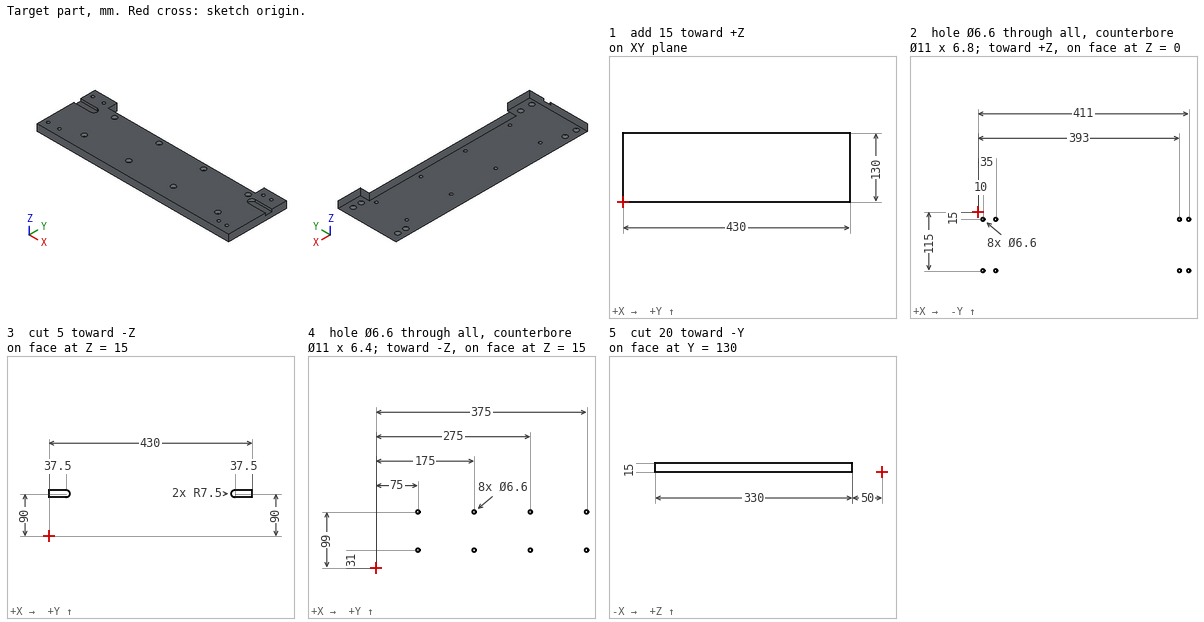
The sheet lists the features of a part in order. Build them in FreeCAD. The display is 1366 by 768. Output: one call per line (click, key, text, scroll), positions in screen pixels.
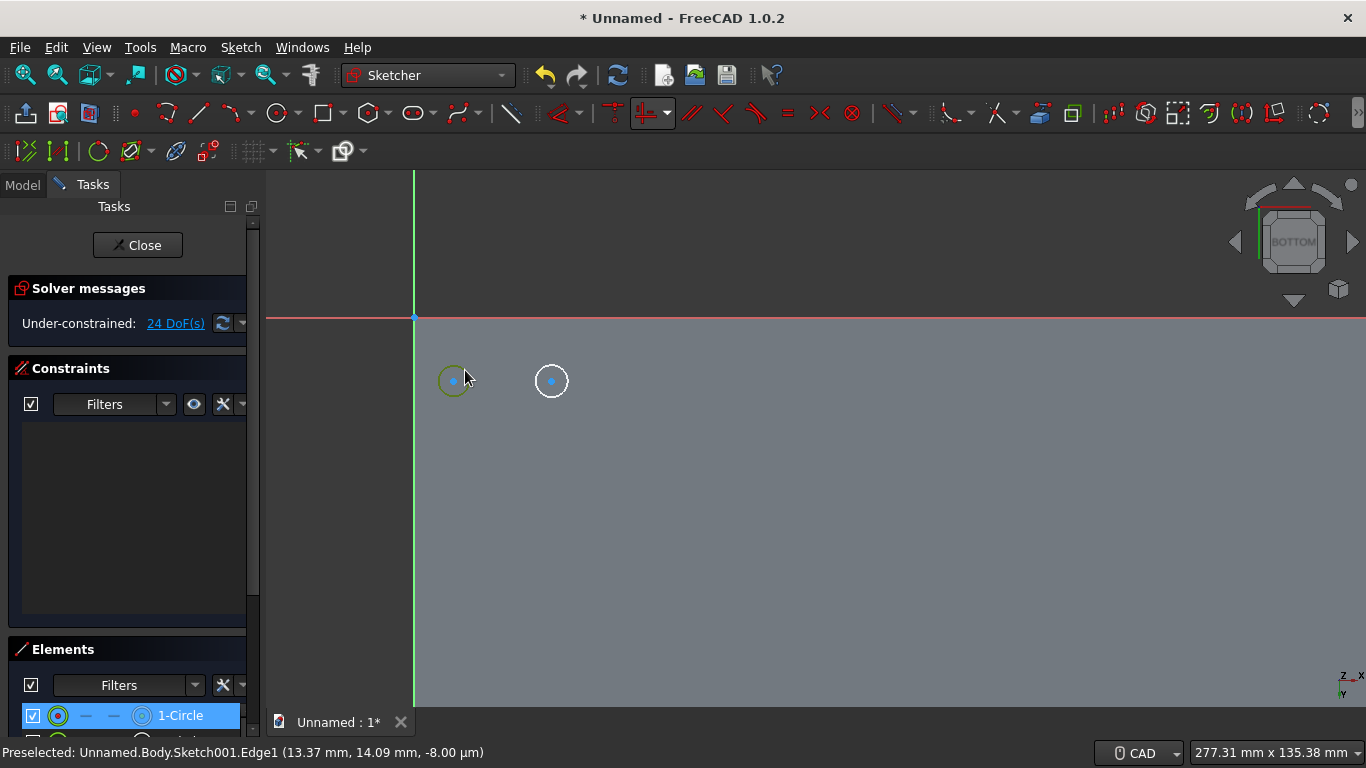
scroll(463, 372, down, 5)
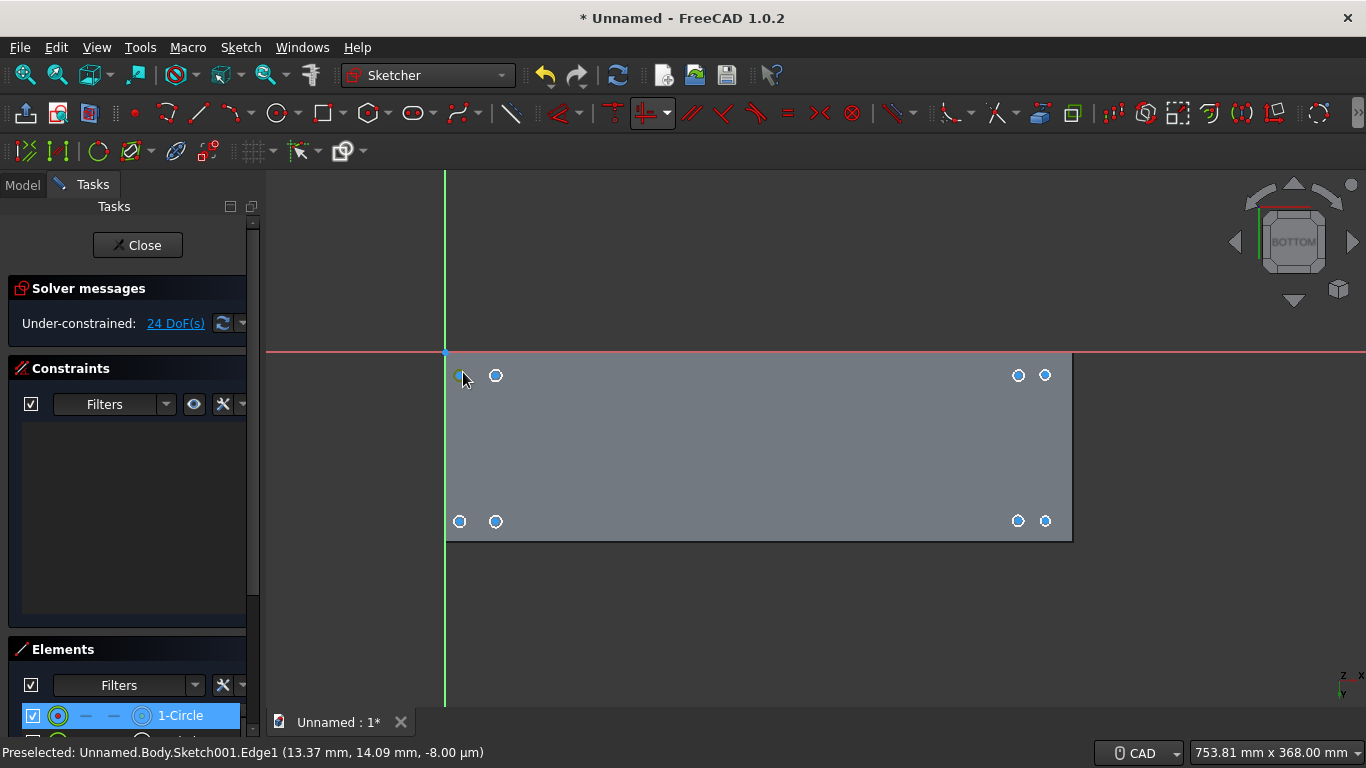
scroll(464, 518, up, 5)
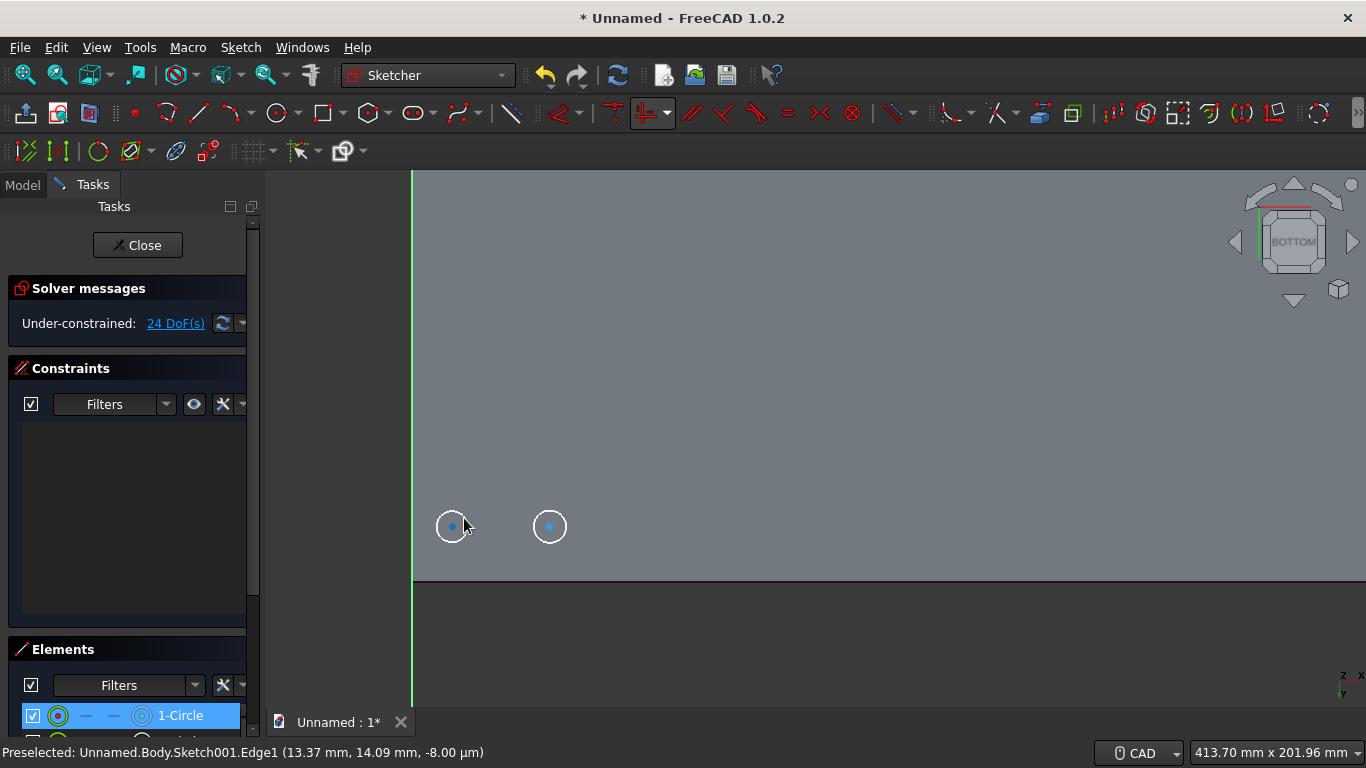
click(463, 516)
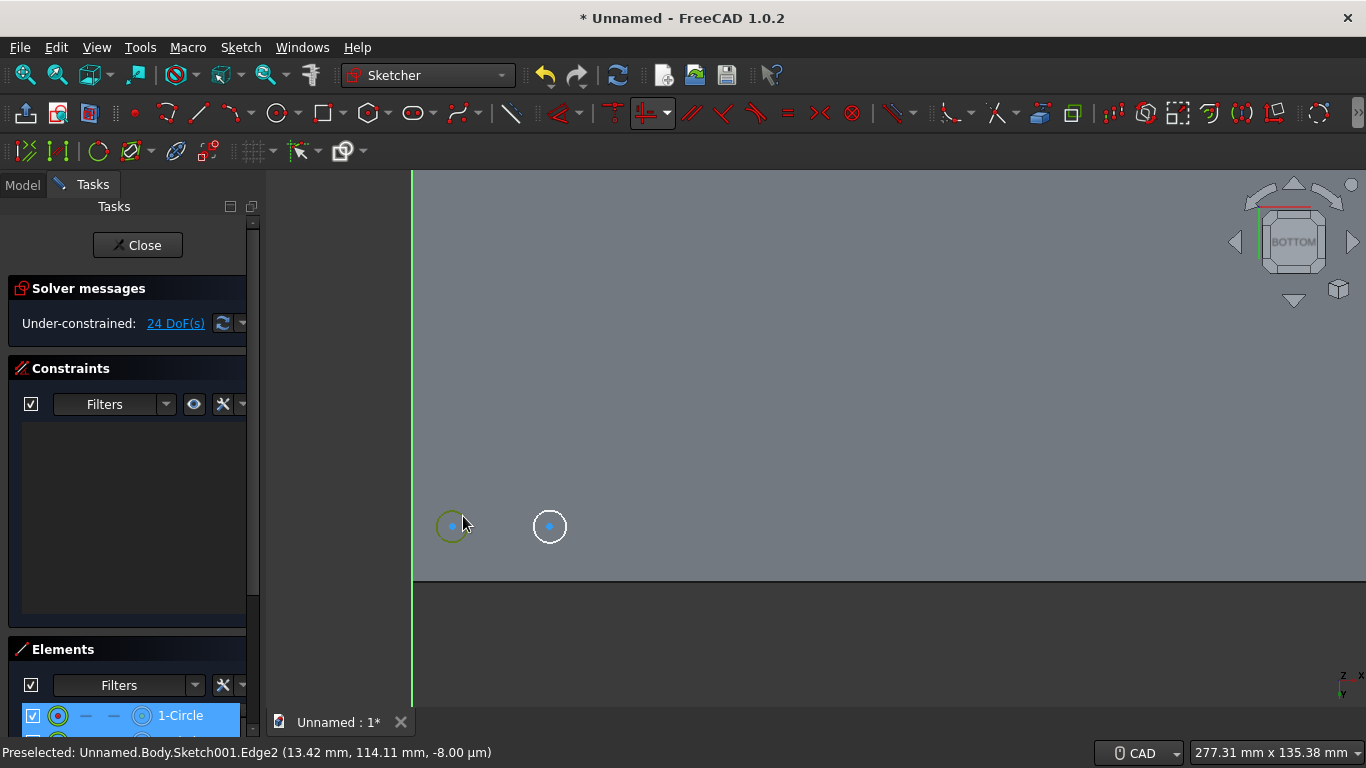
scroll(464, 518, down, 5)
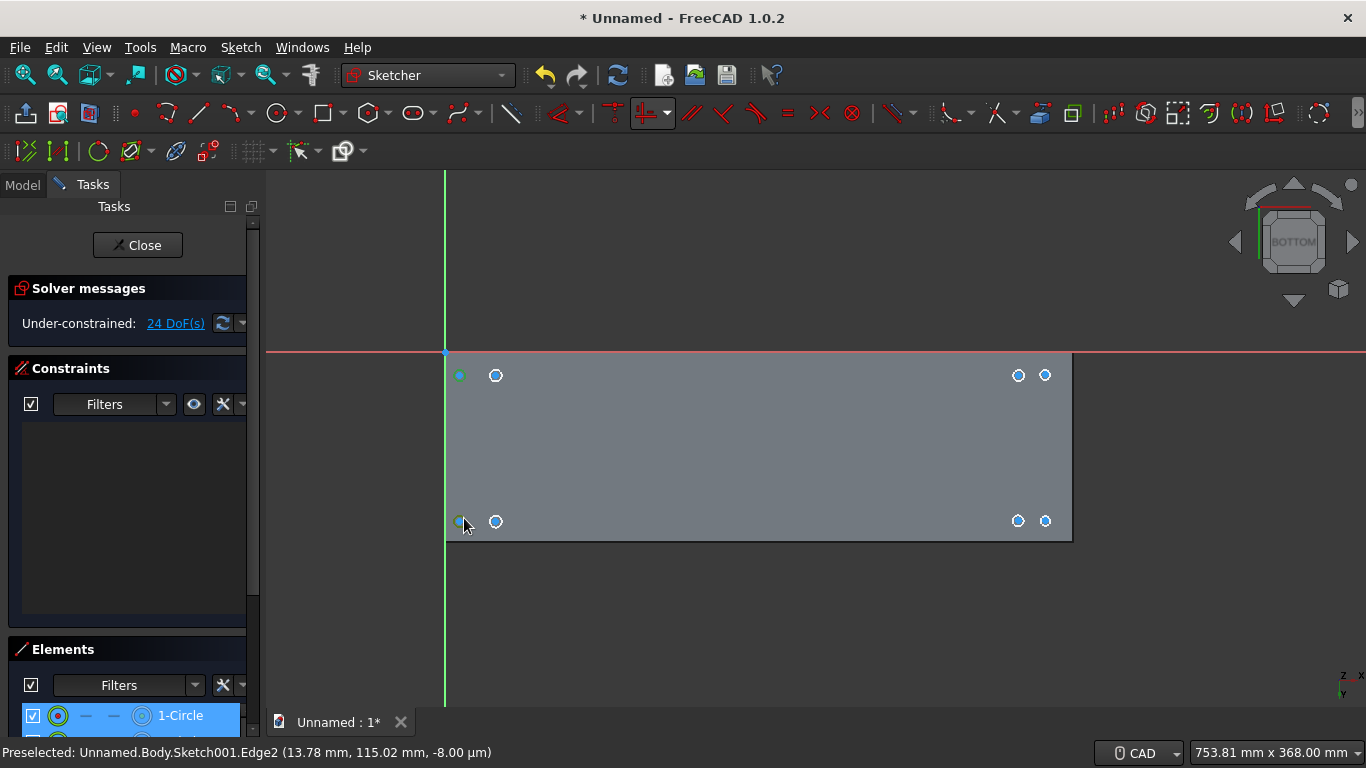
scroll(500, 371, up, 5)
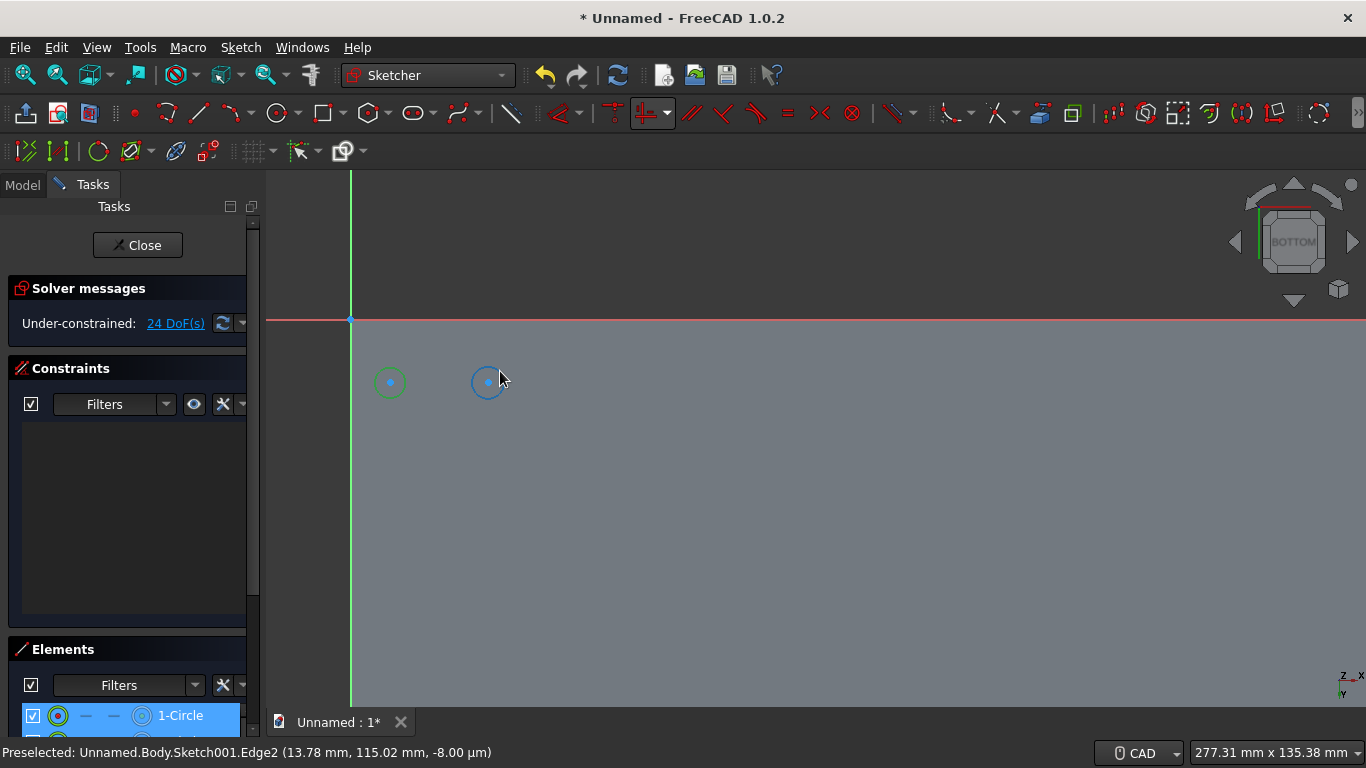
click(499, 372)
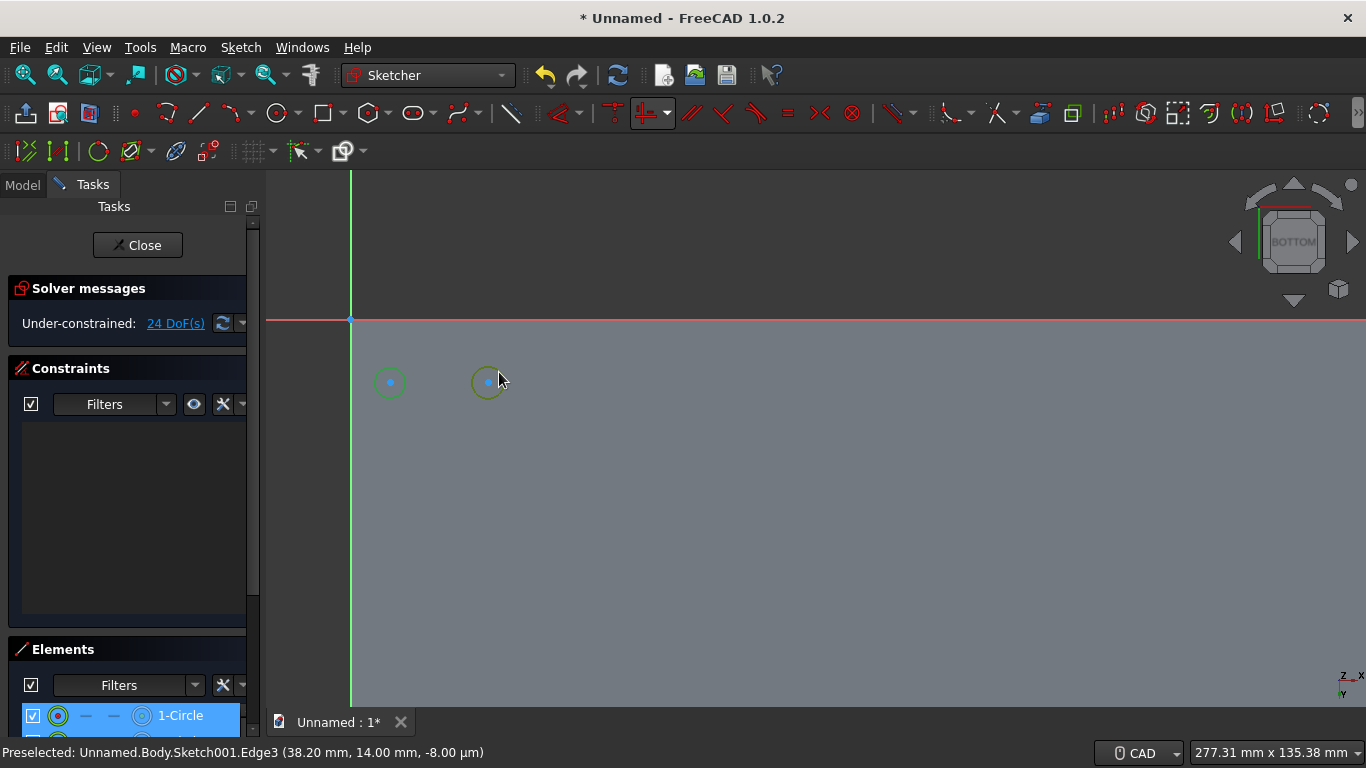
scroll(500, 371, down, 5)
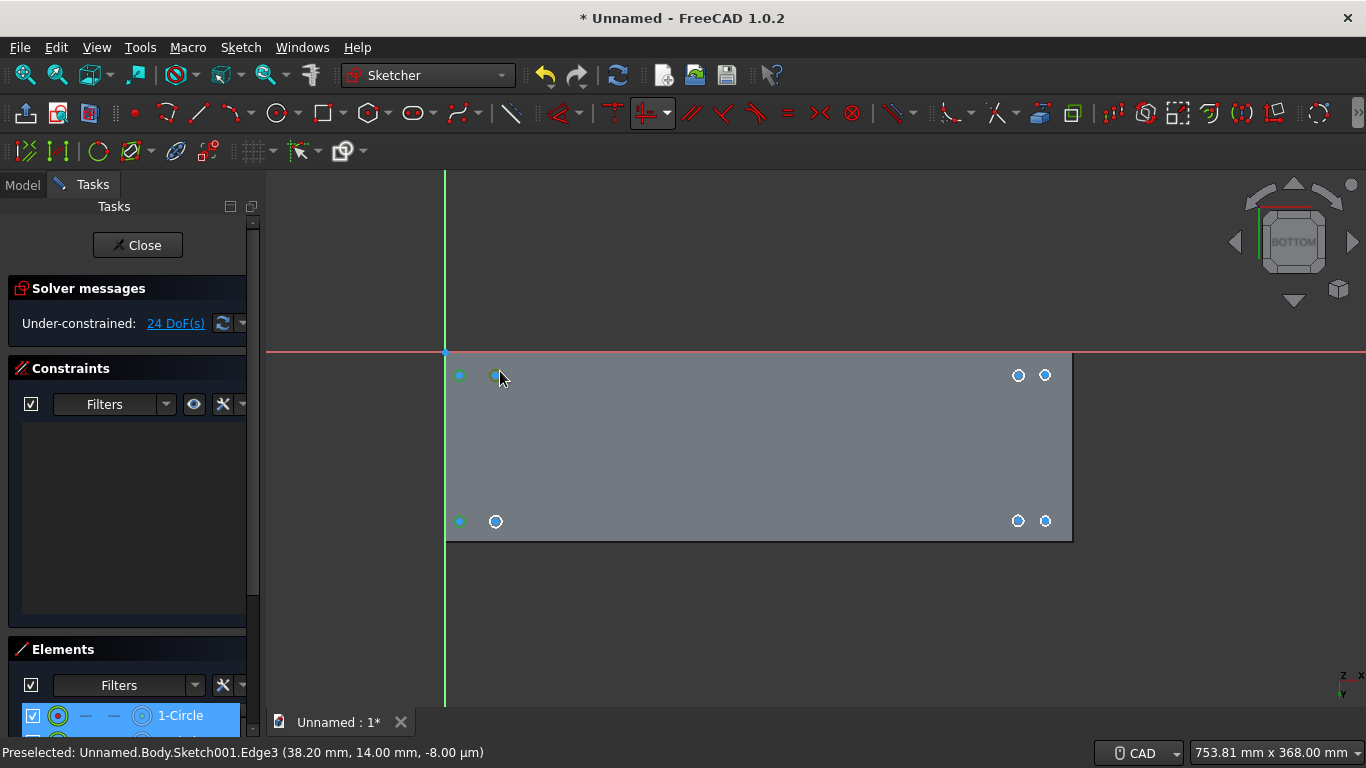
scroll(500, 517, up, 5)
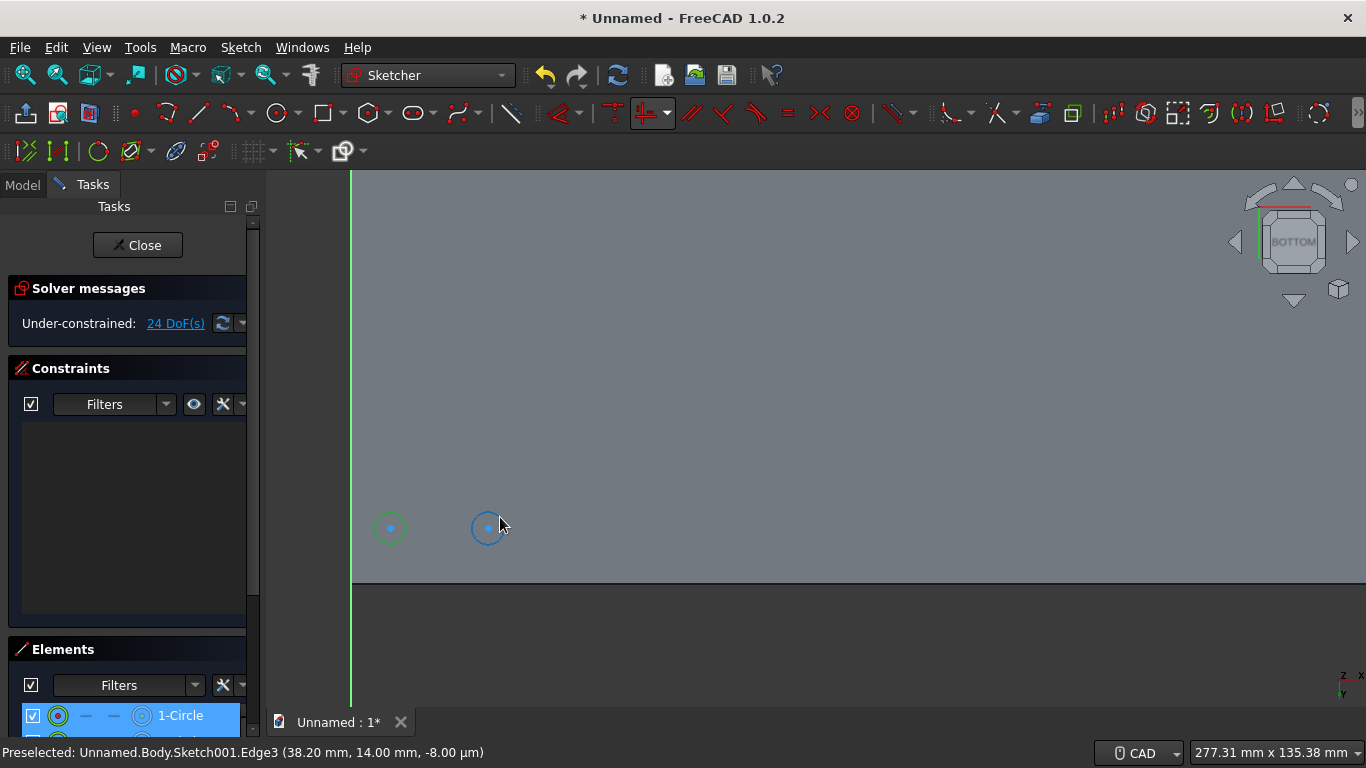
click(499, 517)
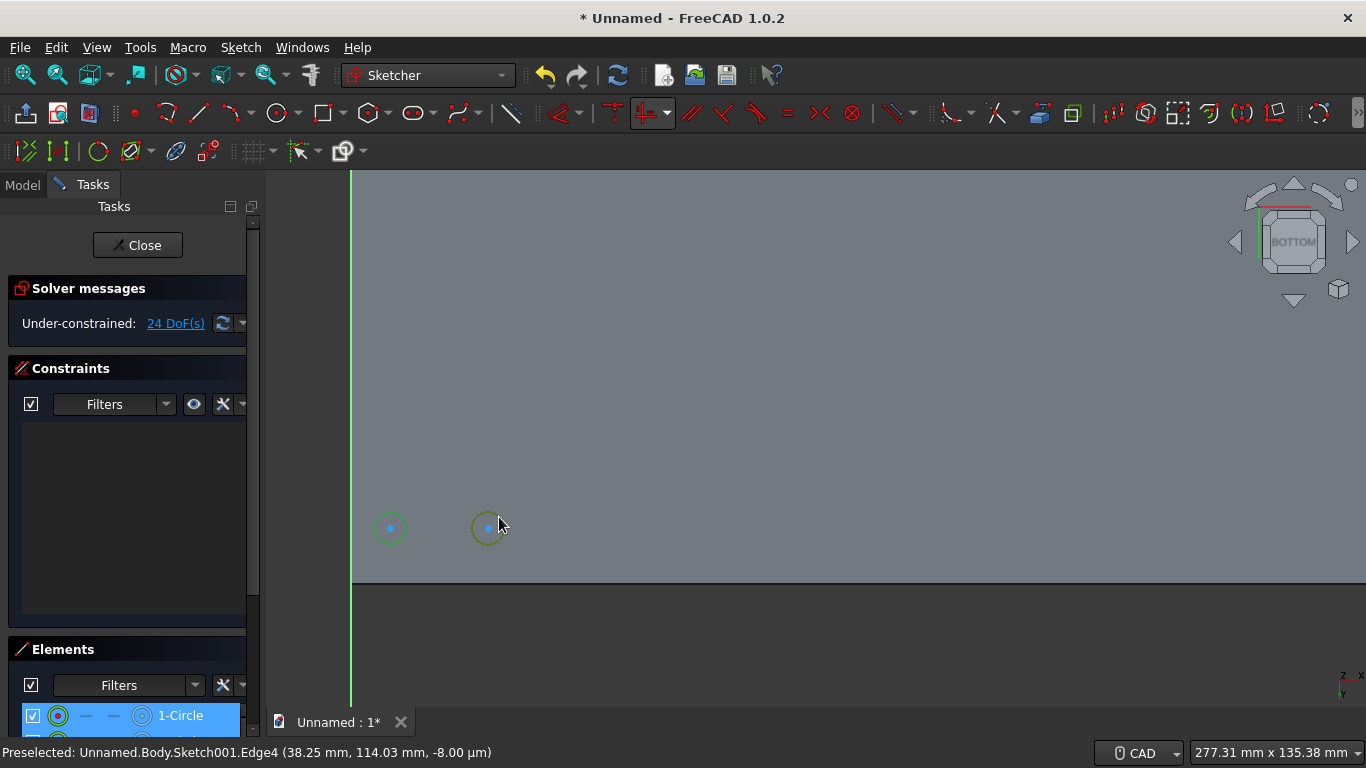
scroll(500, 517, down, 5)